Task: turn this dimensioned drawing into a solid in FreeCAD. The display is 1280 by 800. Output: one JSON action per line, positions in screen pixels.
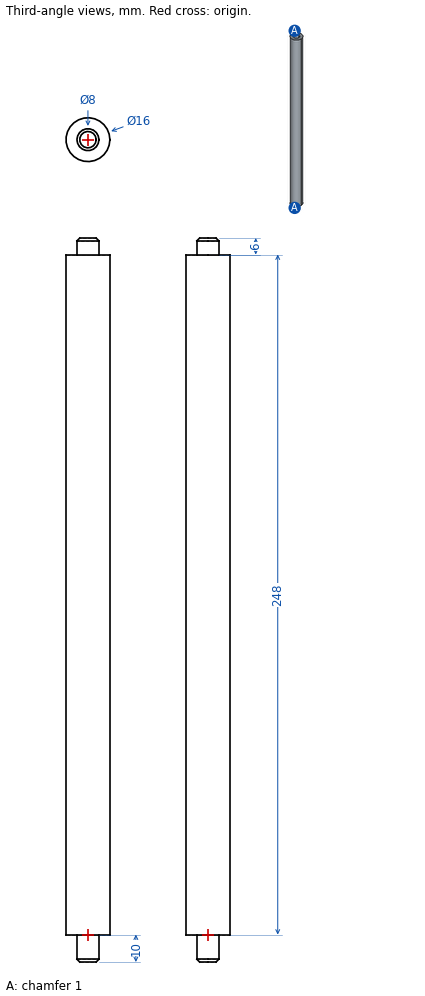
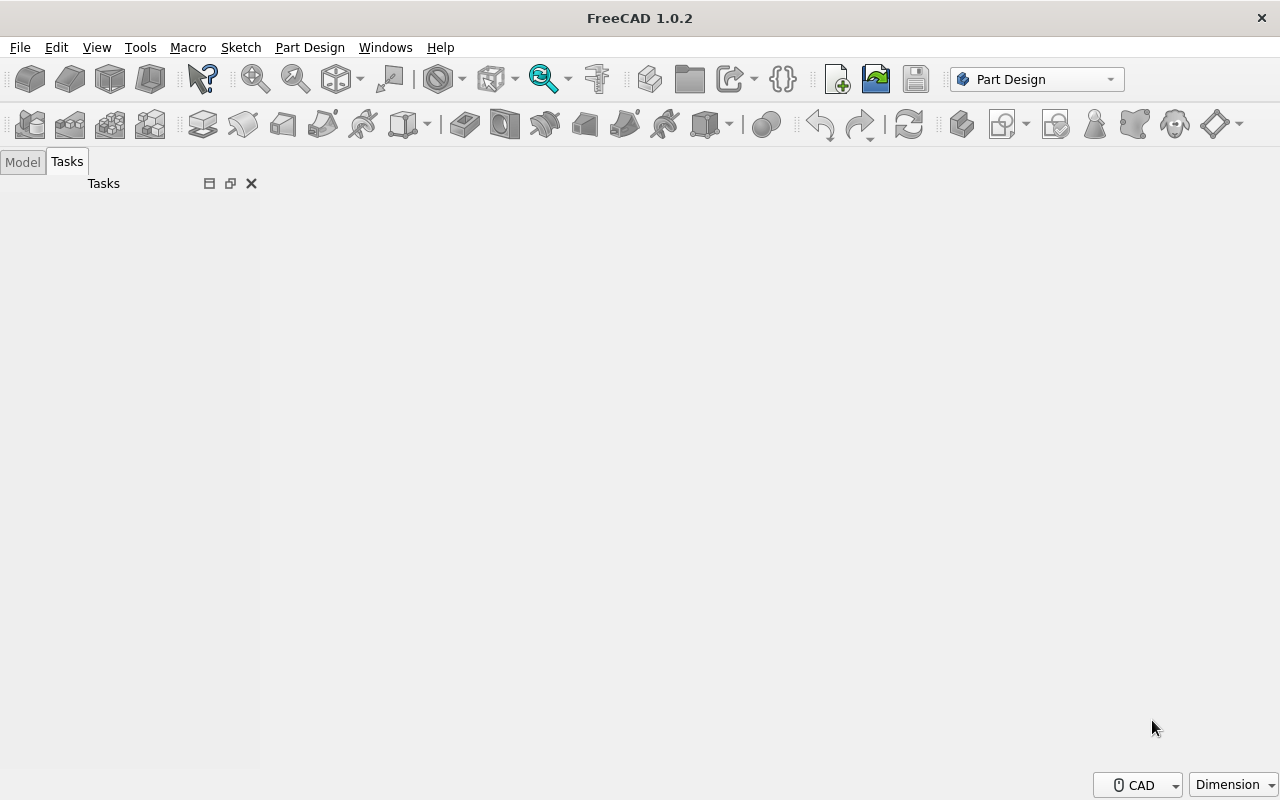
{"action": "key", "text": "ctrl+n"}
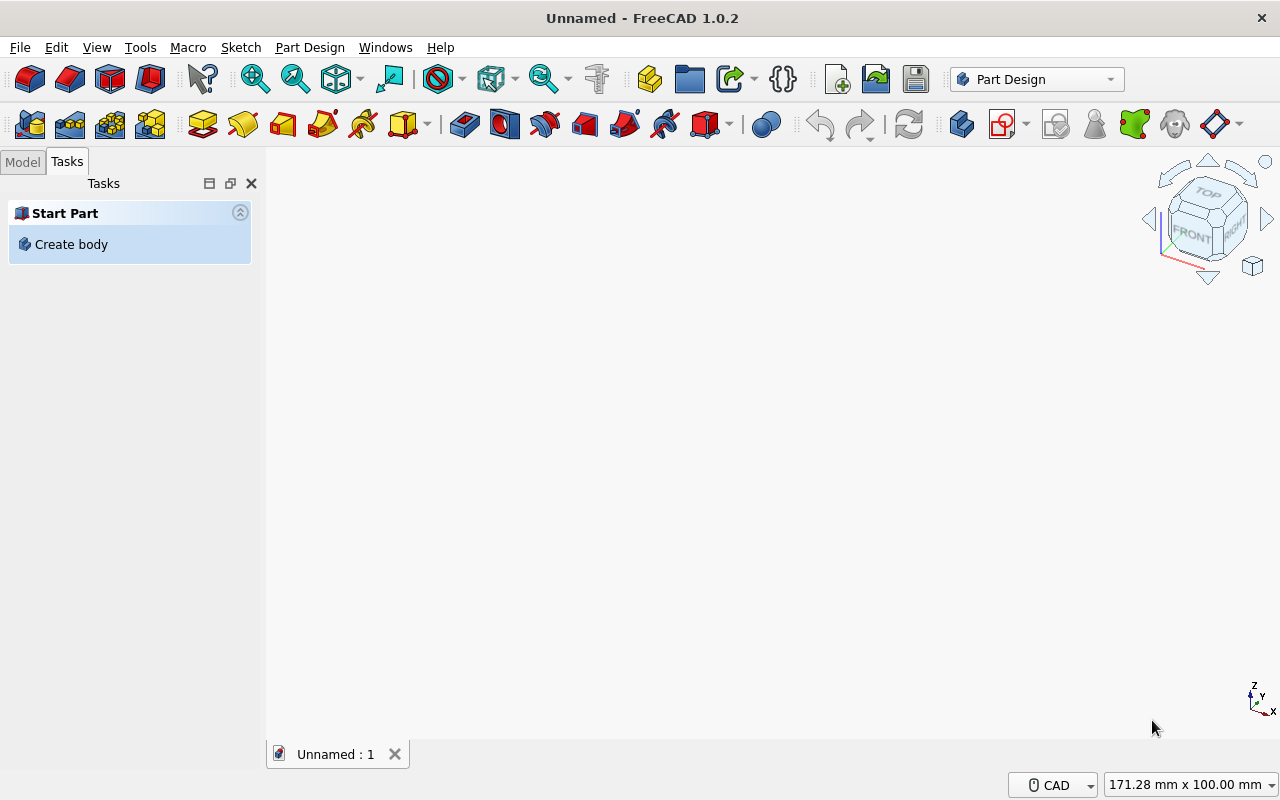
{"action": "left_click", "coordinate": [1002, 124]}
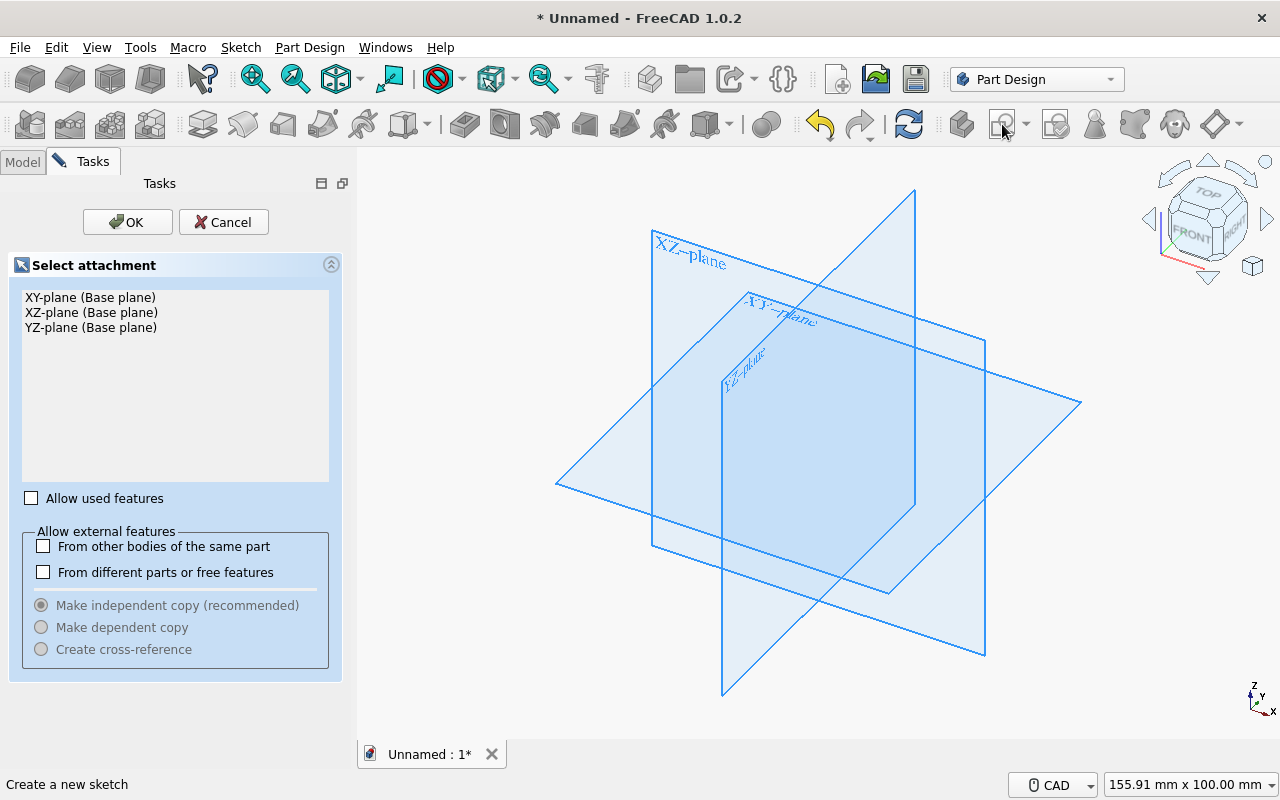
{"action": "left_click", "coordinate": [82, 298]}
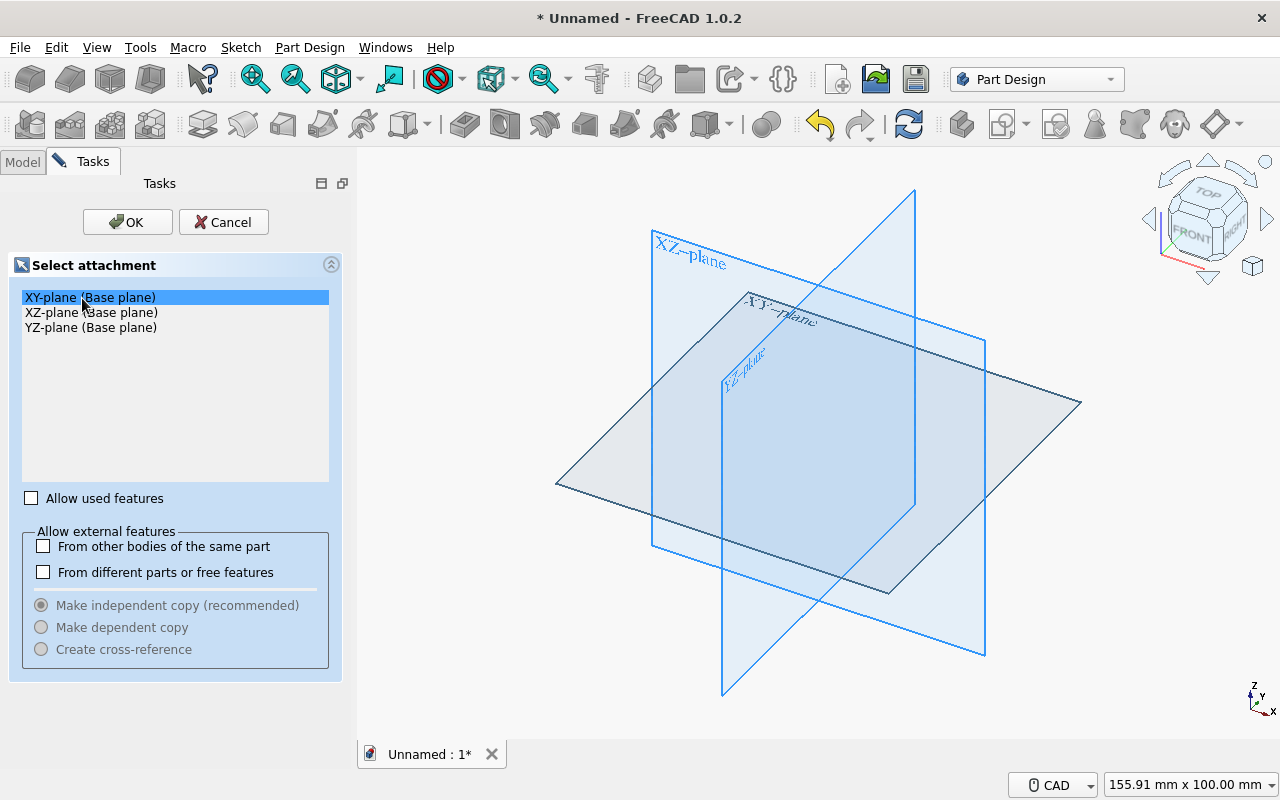
{"action": "left_click", "coordinate": [128, 222]}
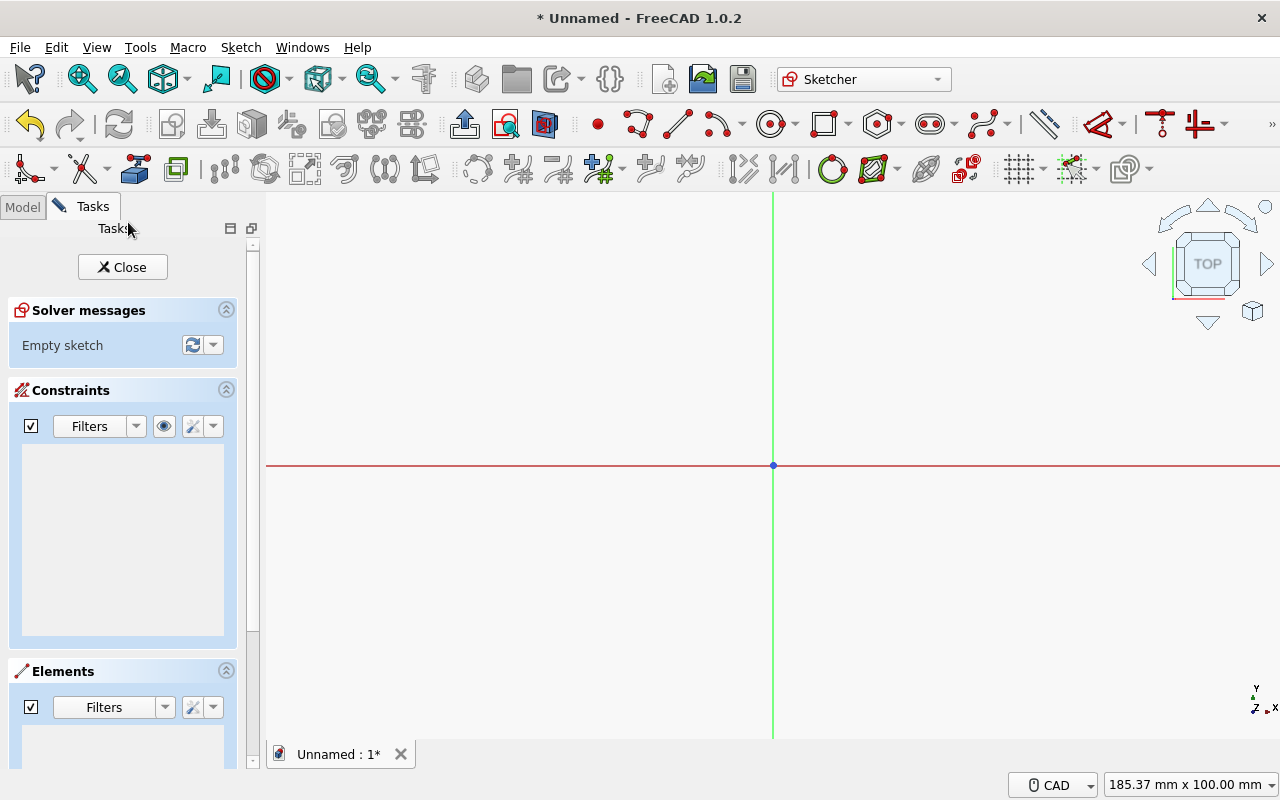
{"action": "scroll", "coordinate": [795, 466], "scroll_direction": "up", "scroll_amount": 7}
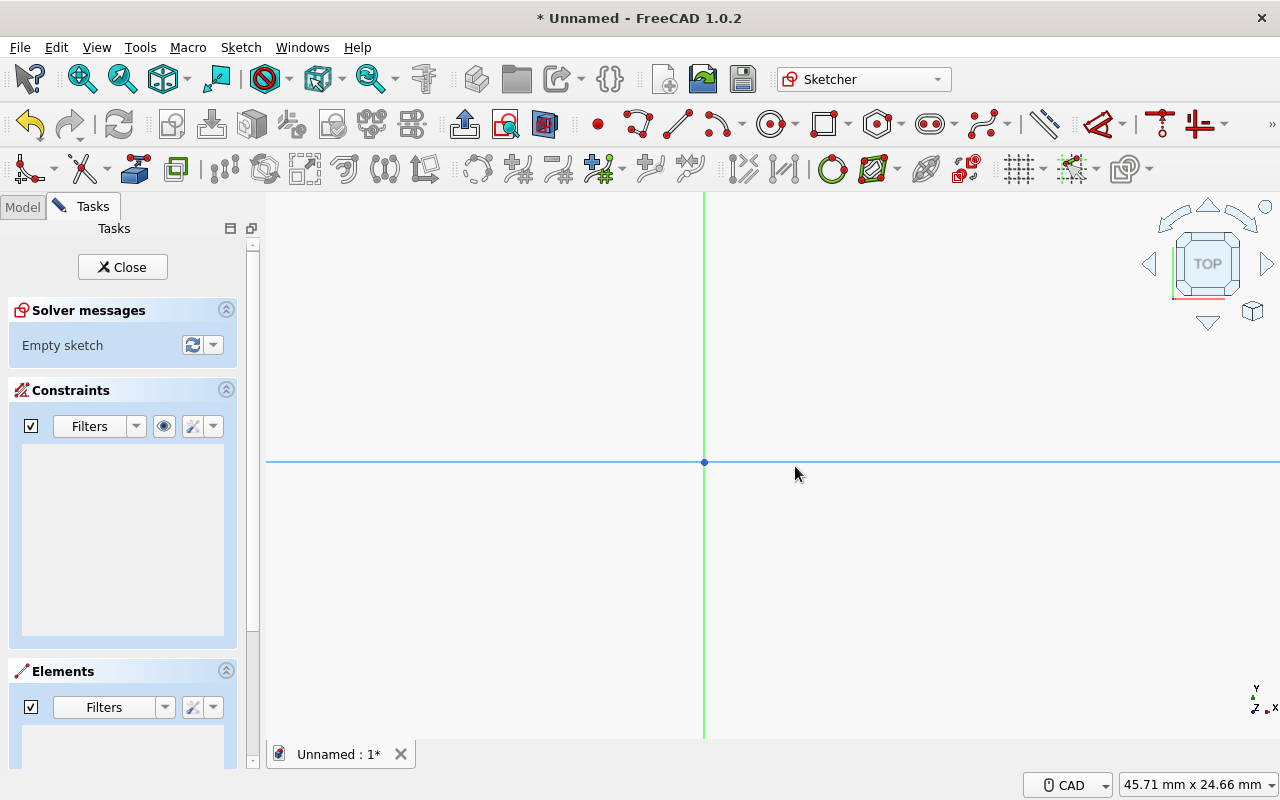
{"action": "key", "text": "g c"}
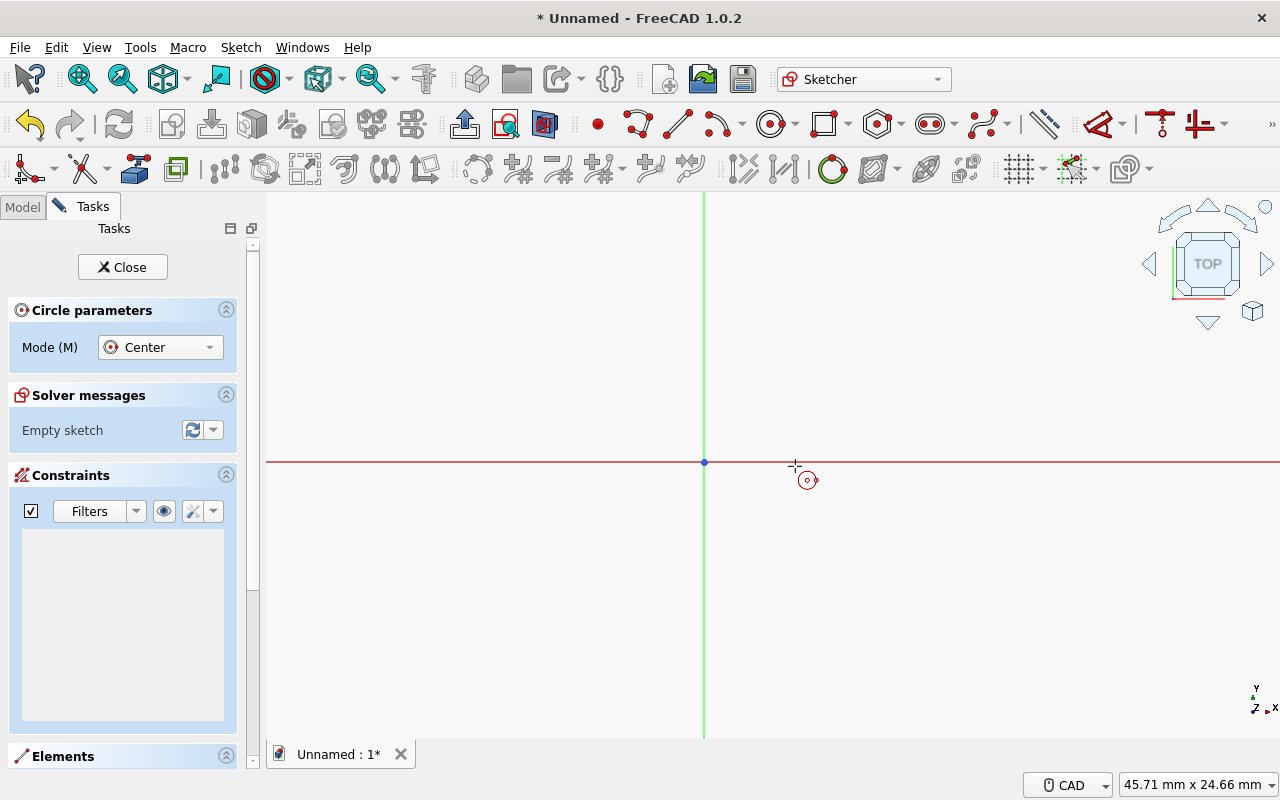
{"action": "left_click", "coordinate": [704, 462]}
{"action": "left_click", "coordinate": [830, 337]}
{"action": "key", "text": "Escape"}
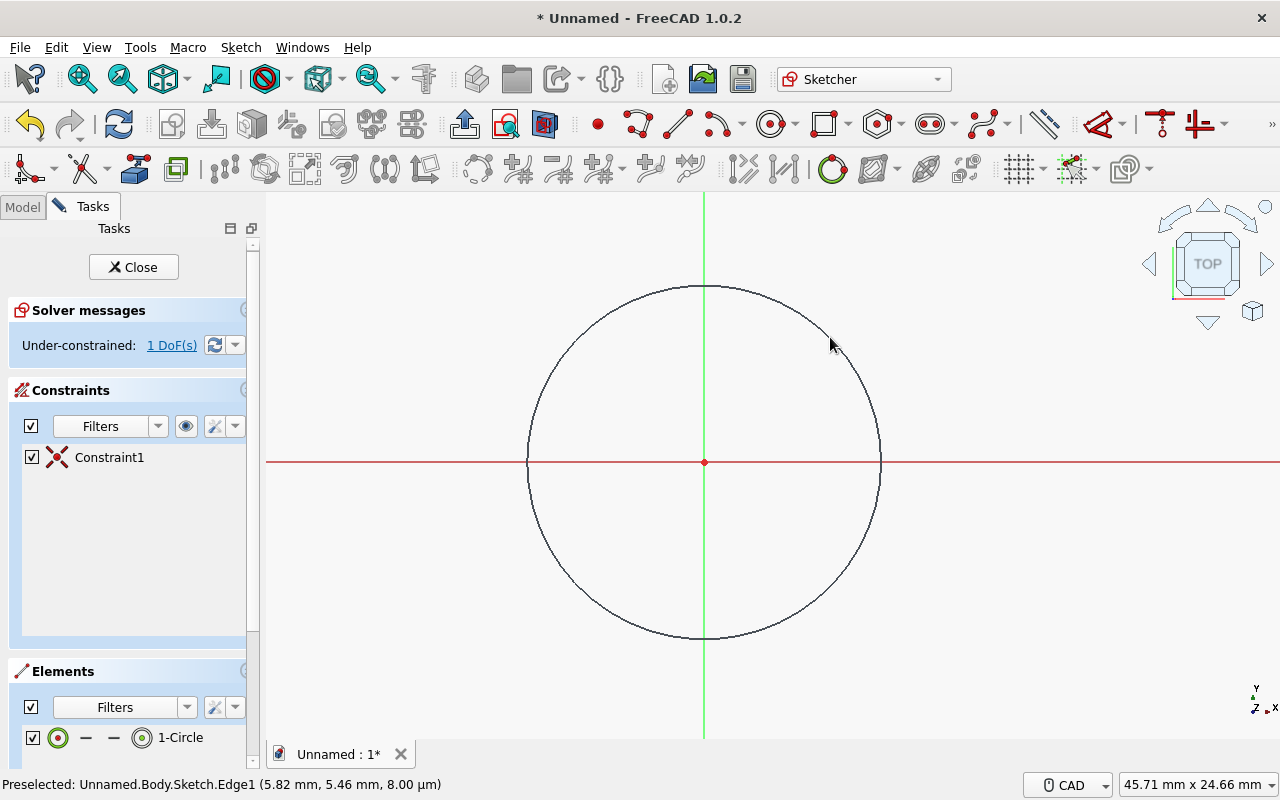
{"action": "key", "text": "d"}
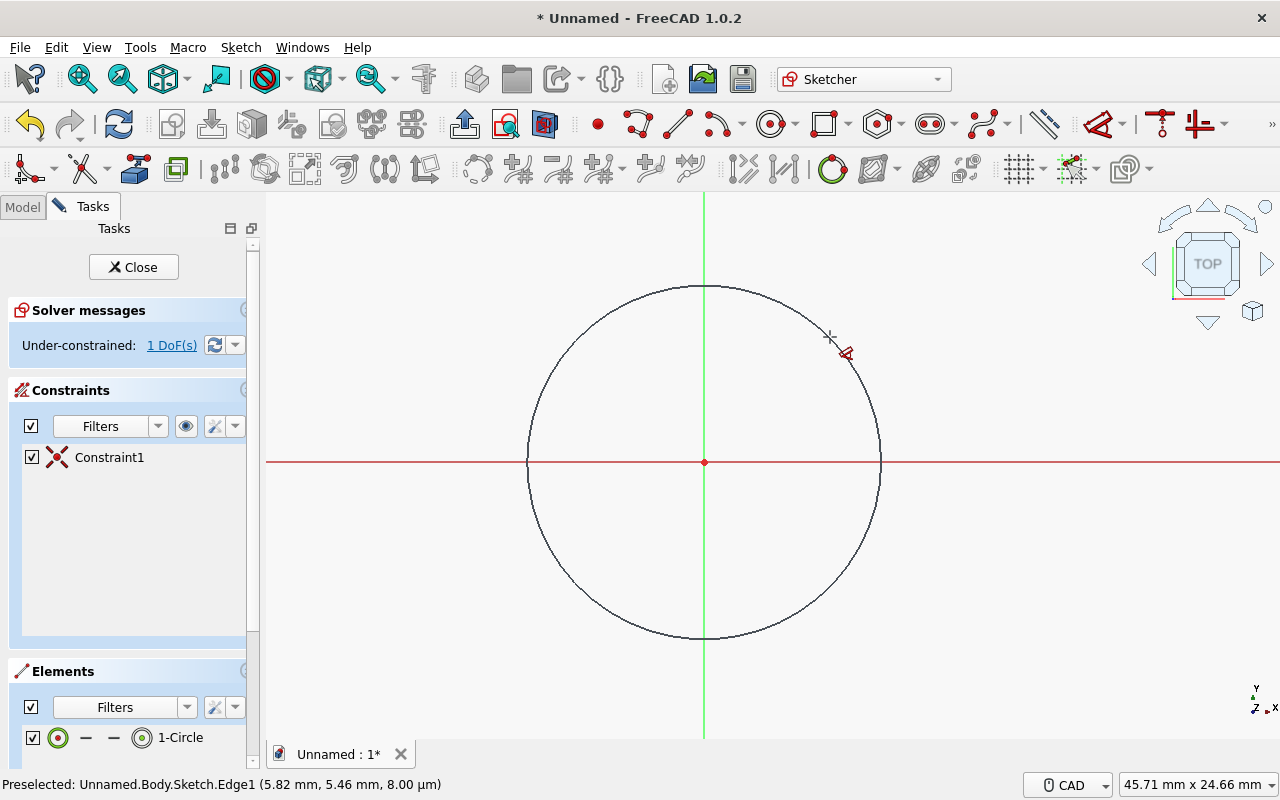
{"action": "left_click", "coordinate": [829, 337]}
{"action": "left_click", "coordinate": [852, 314]}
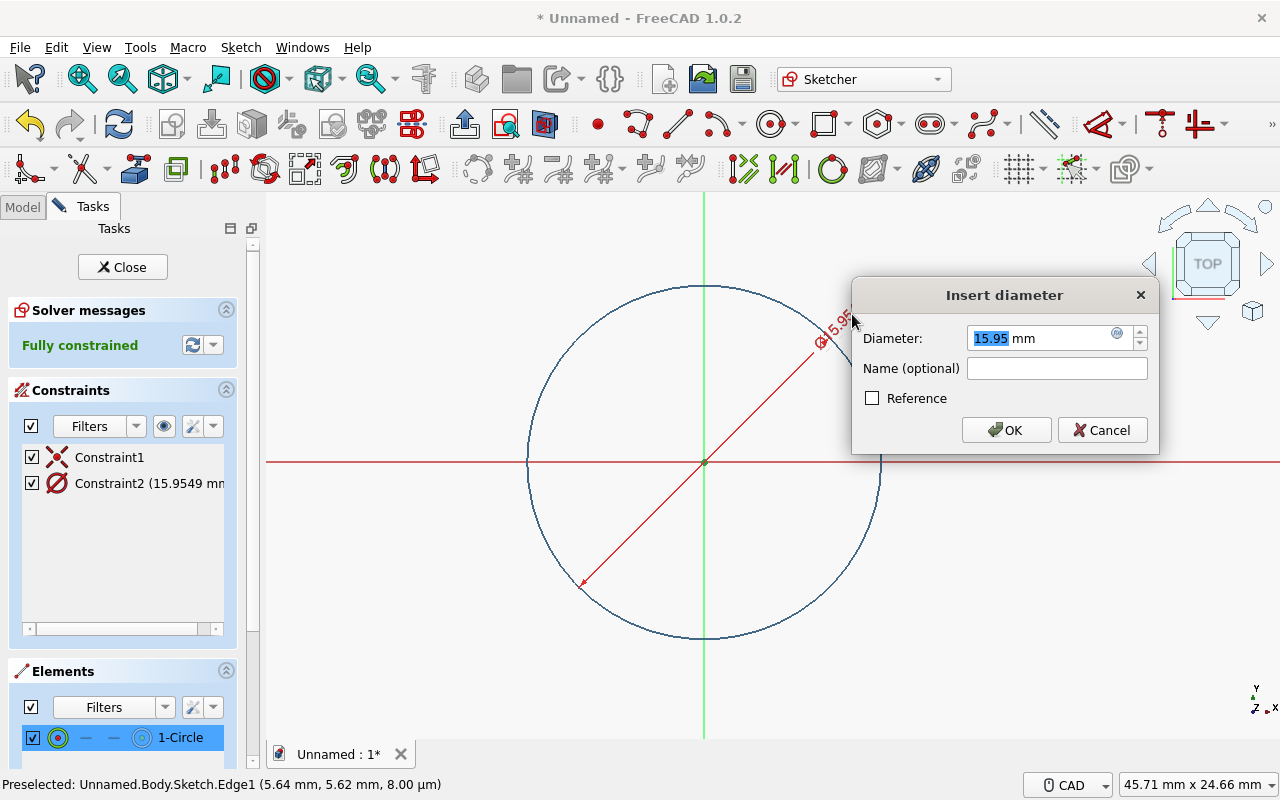
{"action": "type", "text": "16"}
{"action": "key", "text": "Return"}
{"action": "key", "text": "Escape"}